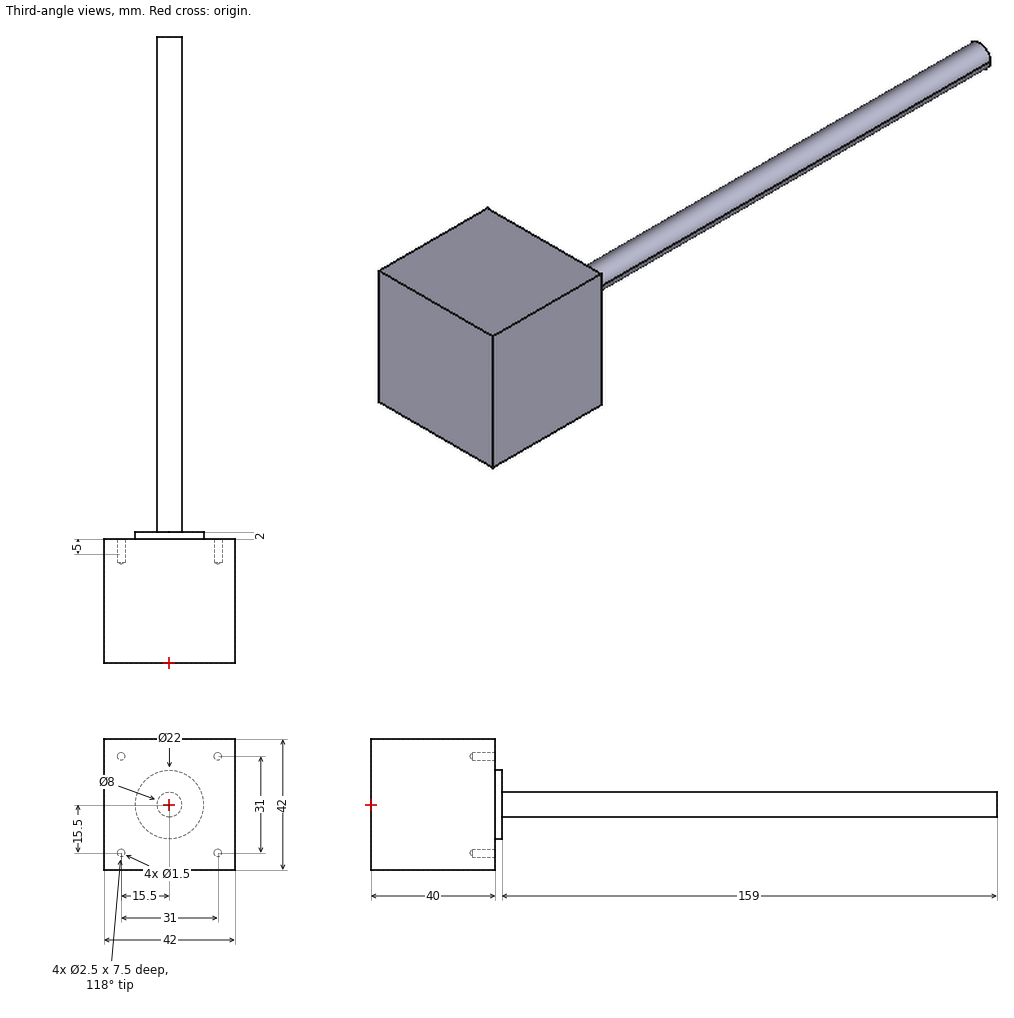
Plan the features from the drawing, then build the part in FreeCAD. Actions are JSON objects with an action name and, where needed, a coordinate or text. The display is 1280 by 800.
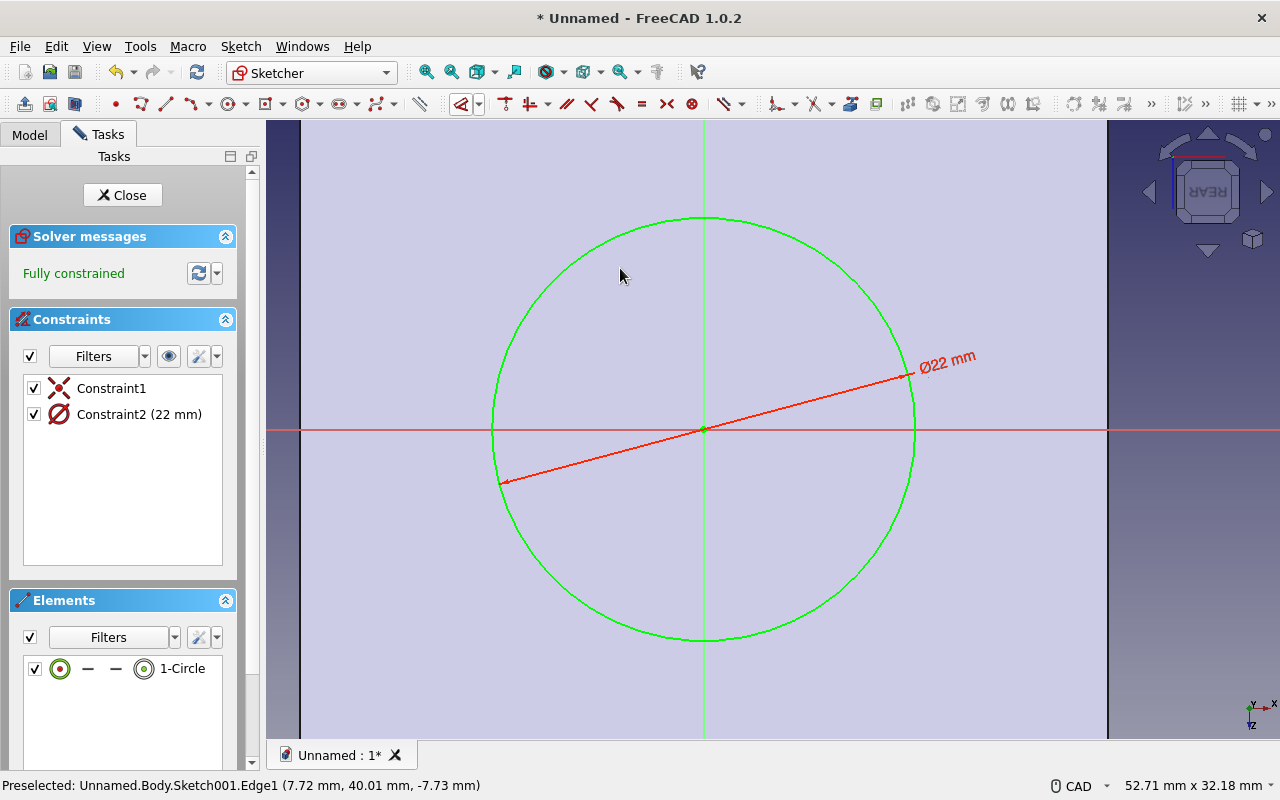
{"action": "left_click", "coordinate": [123, 195]}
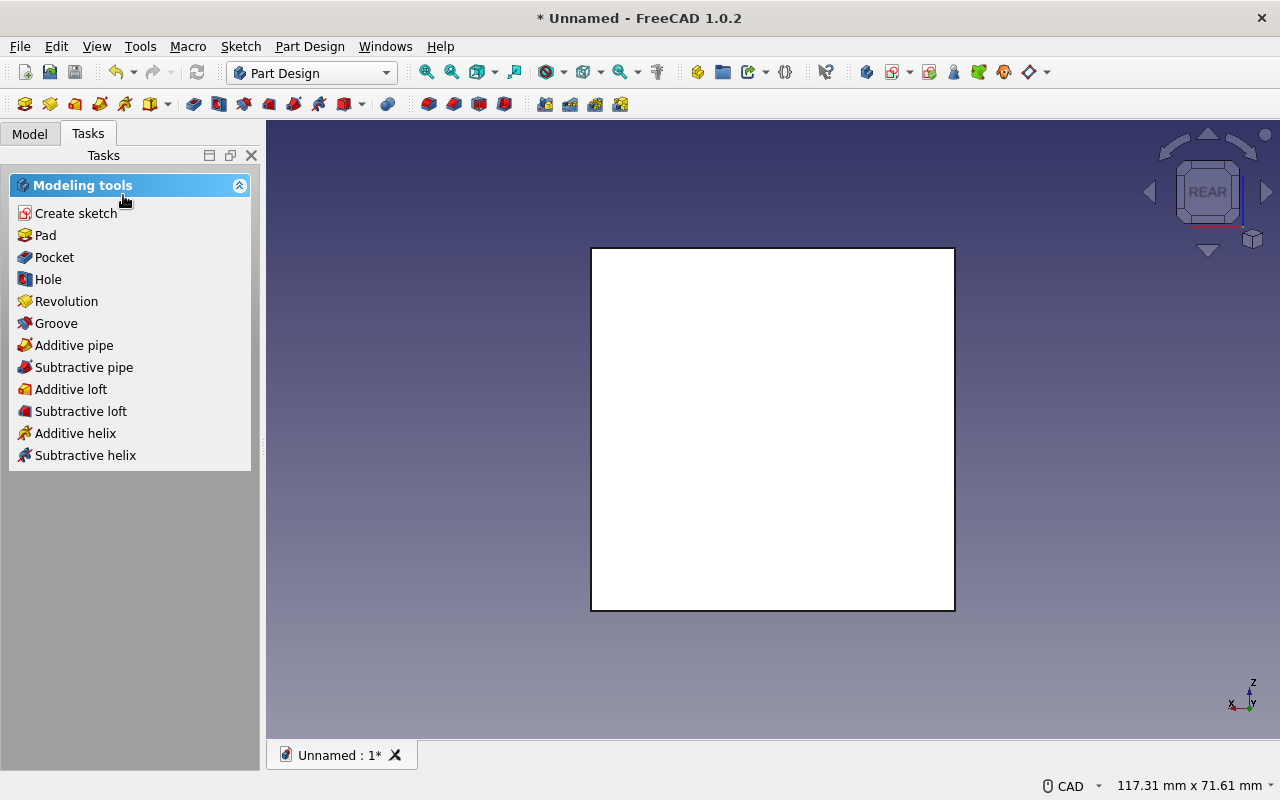
{"action": "left_click", "coordinate": [25, 104]}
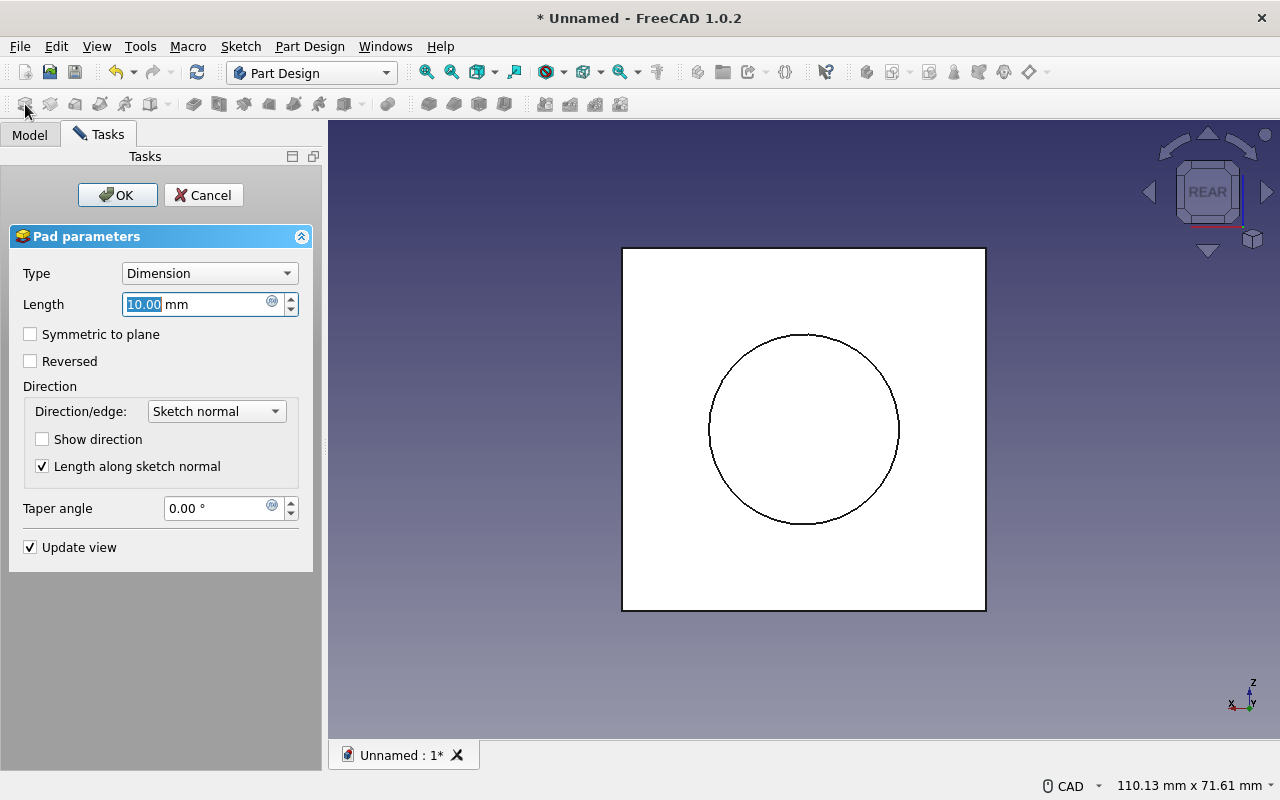
{"action": "type", "text": "2"}
{"action": "key", "text": "Tab"}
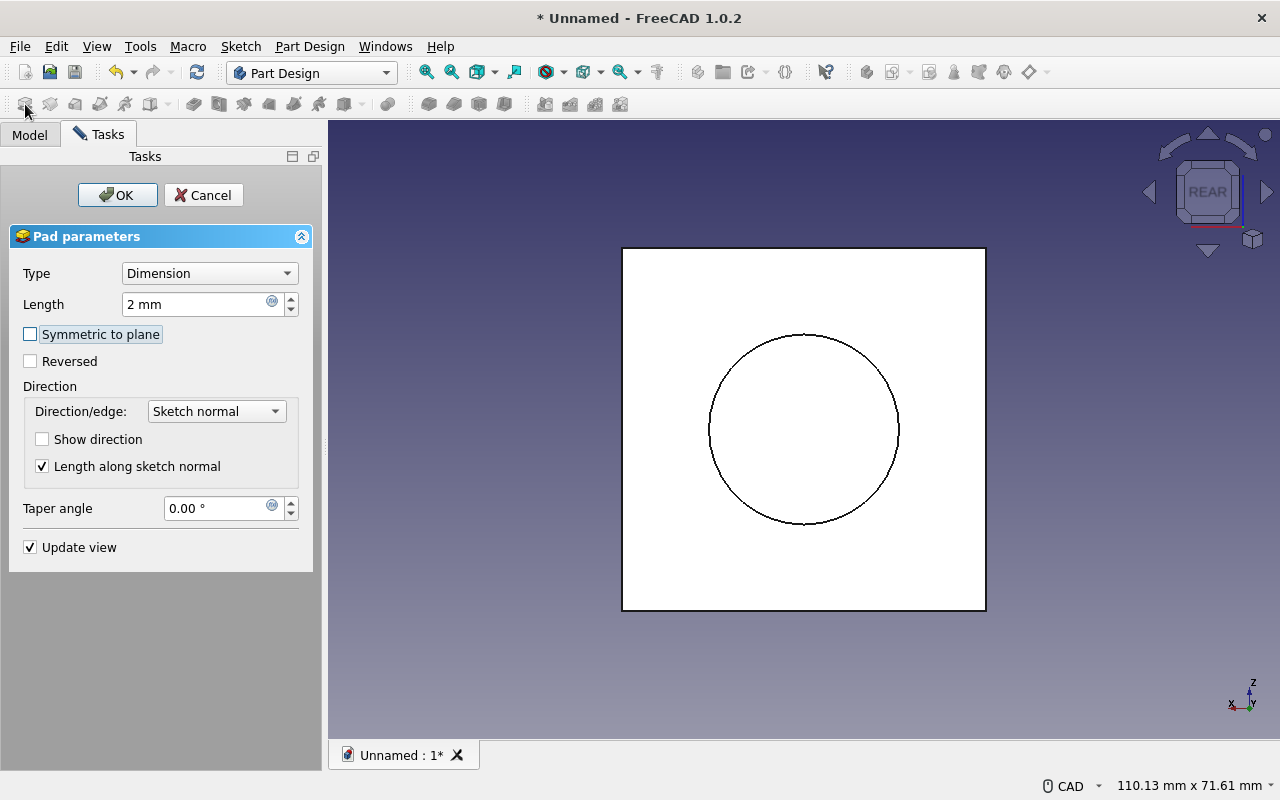
{"action": "left_click", "coordinate": [118, 195]}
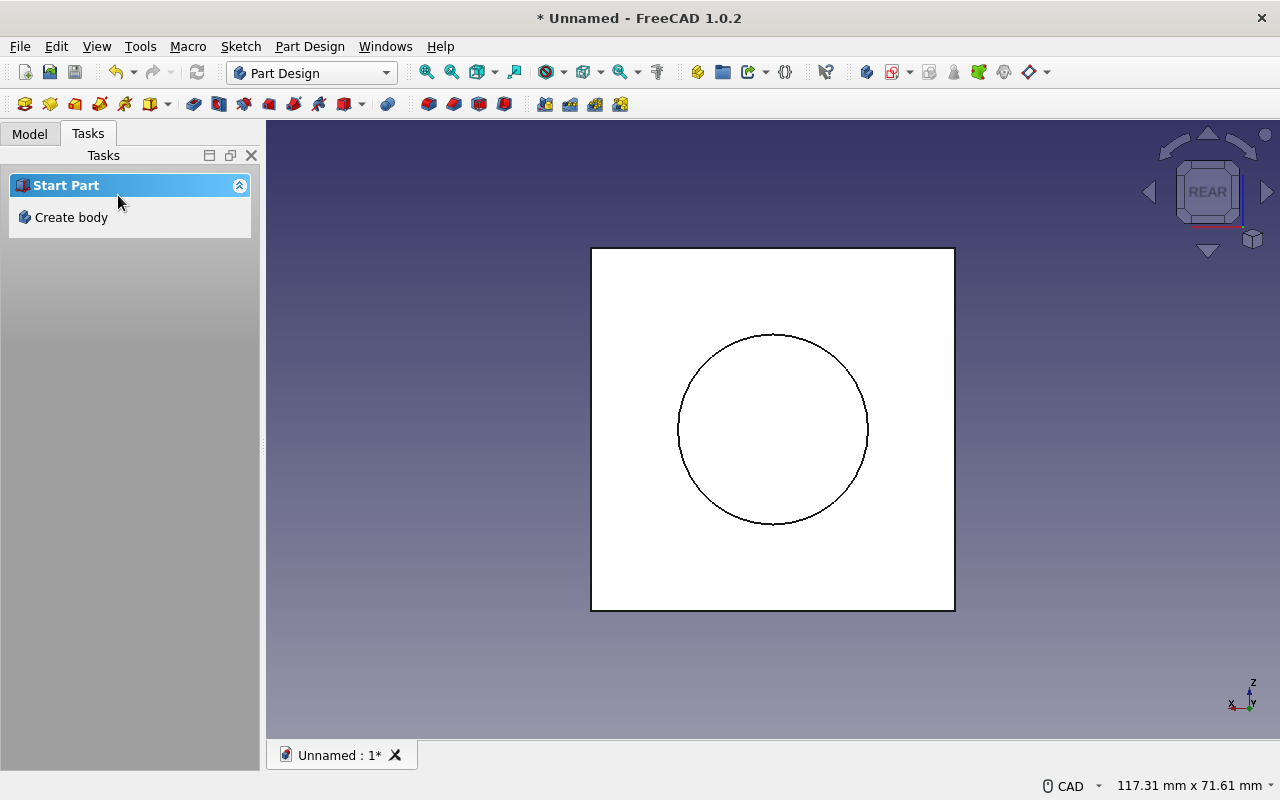
{"action": "left_click", "coordinate": [773, 429]}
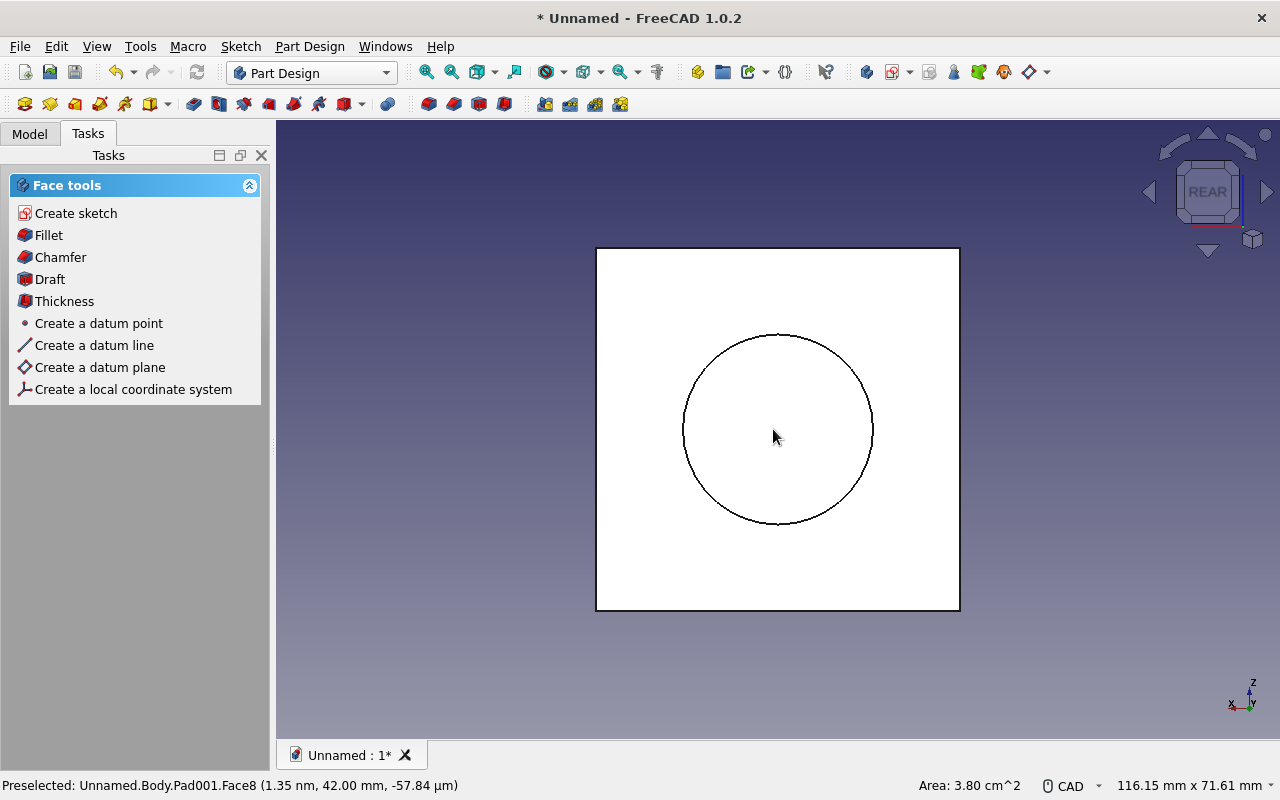
{"action": "left_click", "coordinate": [892, 72]}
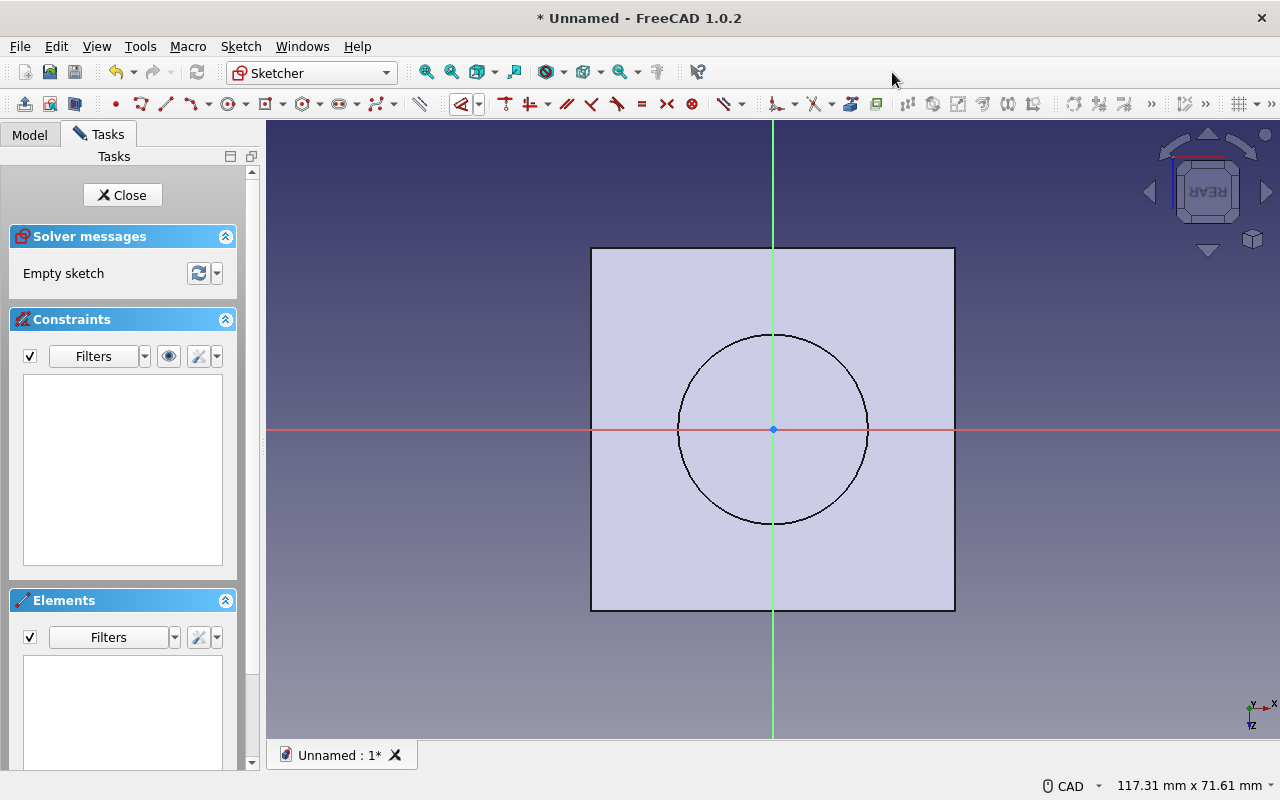
{"action": "scroll", "coordinate": [787, 429], "scroll_direction": "up", "scroll_amount": 9}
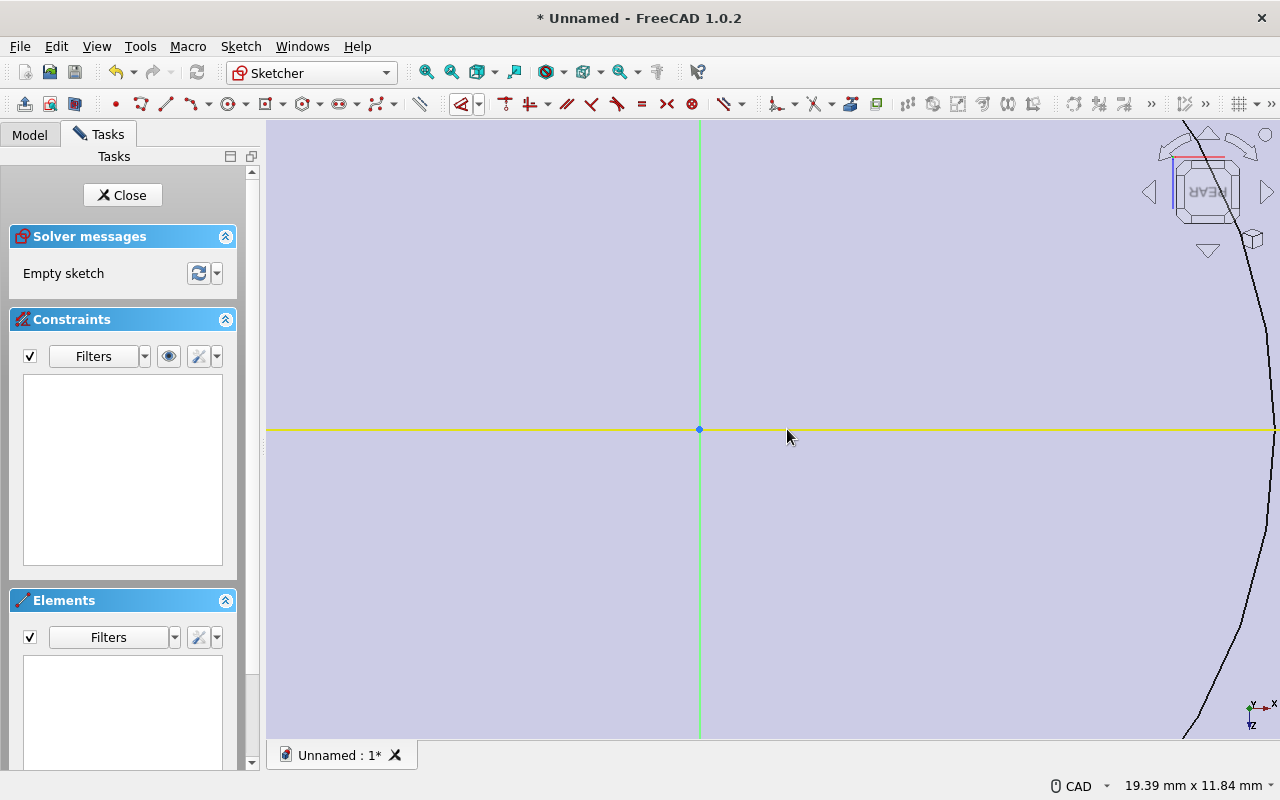
{"action": "key", "text": "g c"}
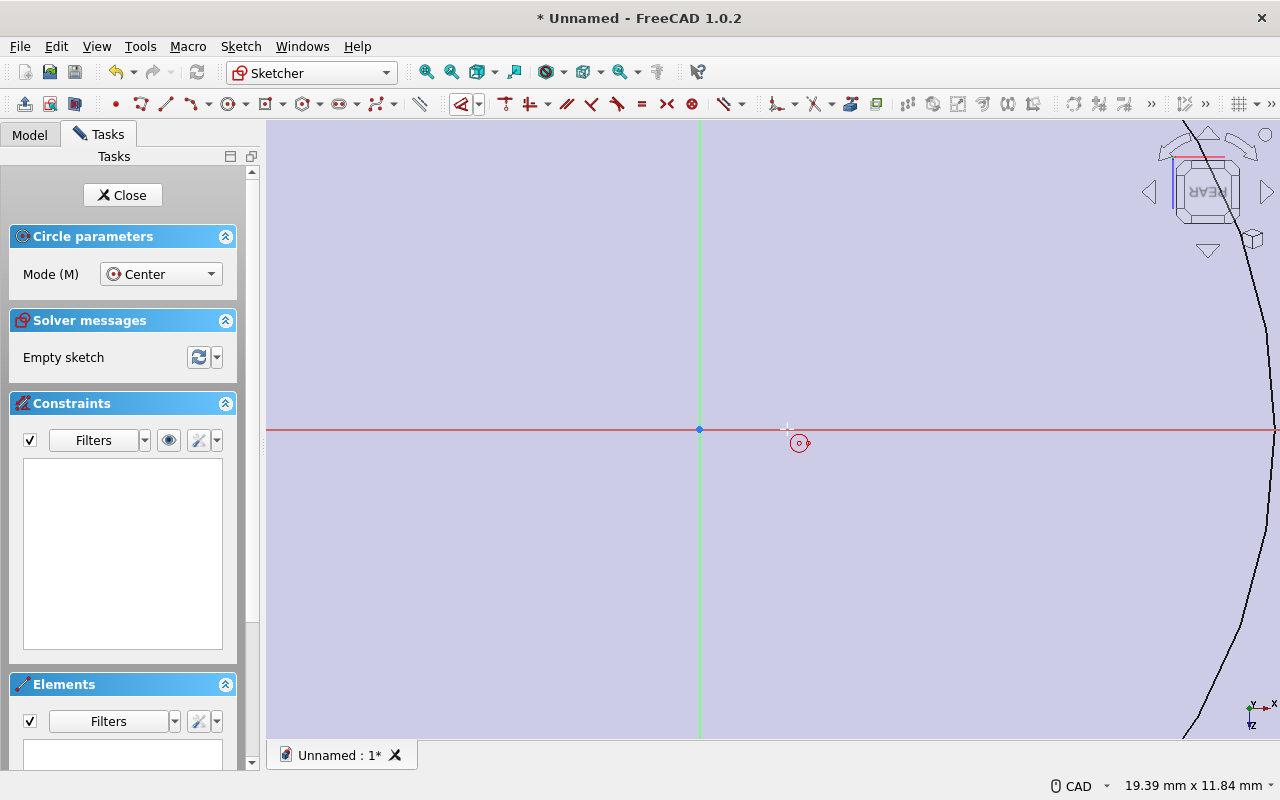
{"action": "left_click", "coordinate": [700, 429]}
{"action": "left_click", "coordinate": [848, 282]}
{"action": "key", "text": "Escape"}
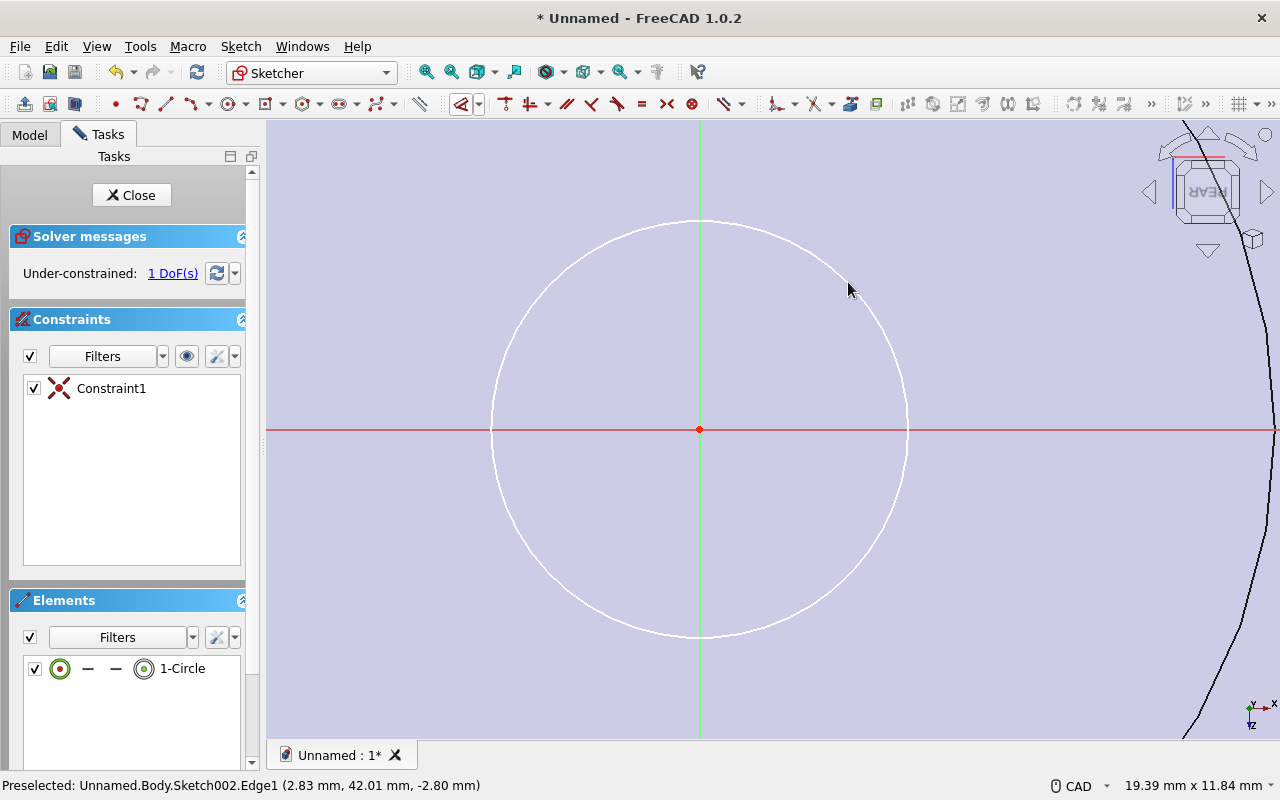
{"action": "left_click", "coordinate": [847, 282]}